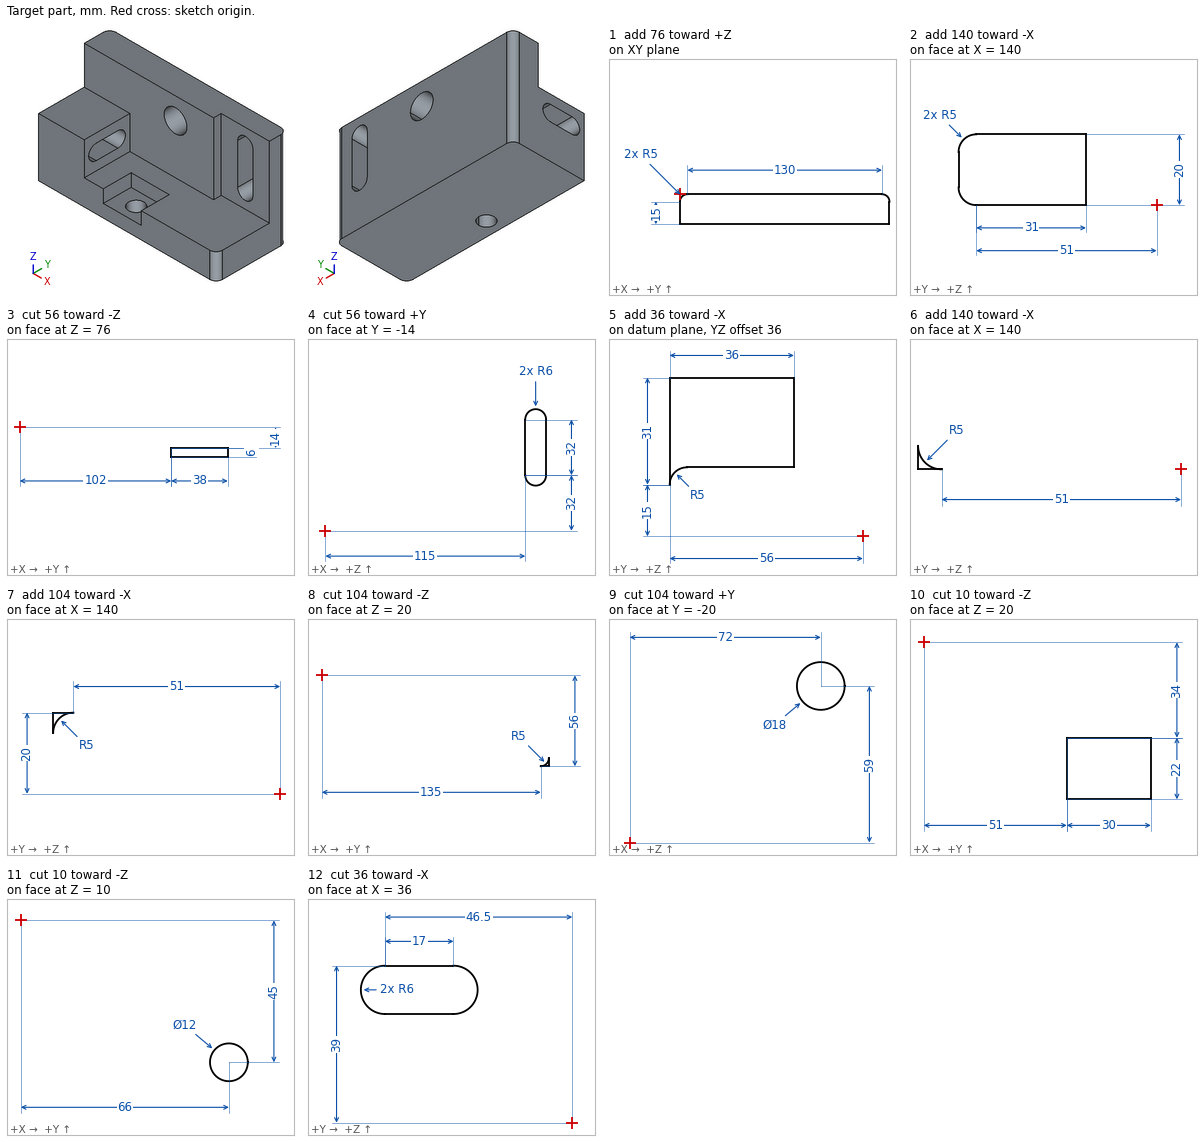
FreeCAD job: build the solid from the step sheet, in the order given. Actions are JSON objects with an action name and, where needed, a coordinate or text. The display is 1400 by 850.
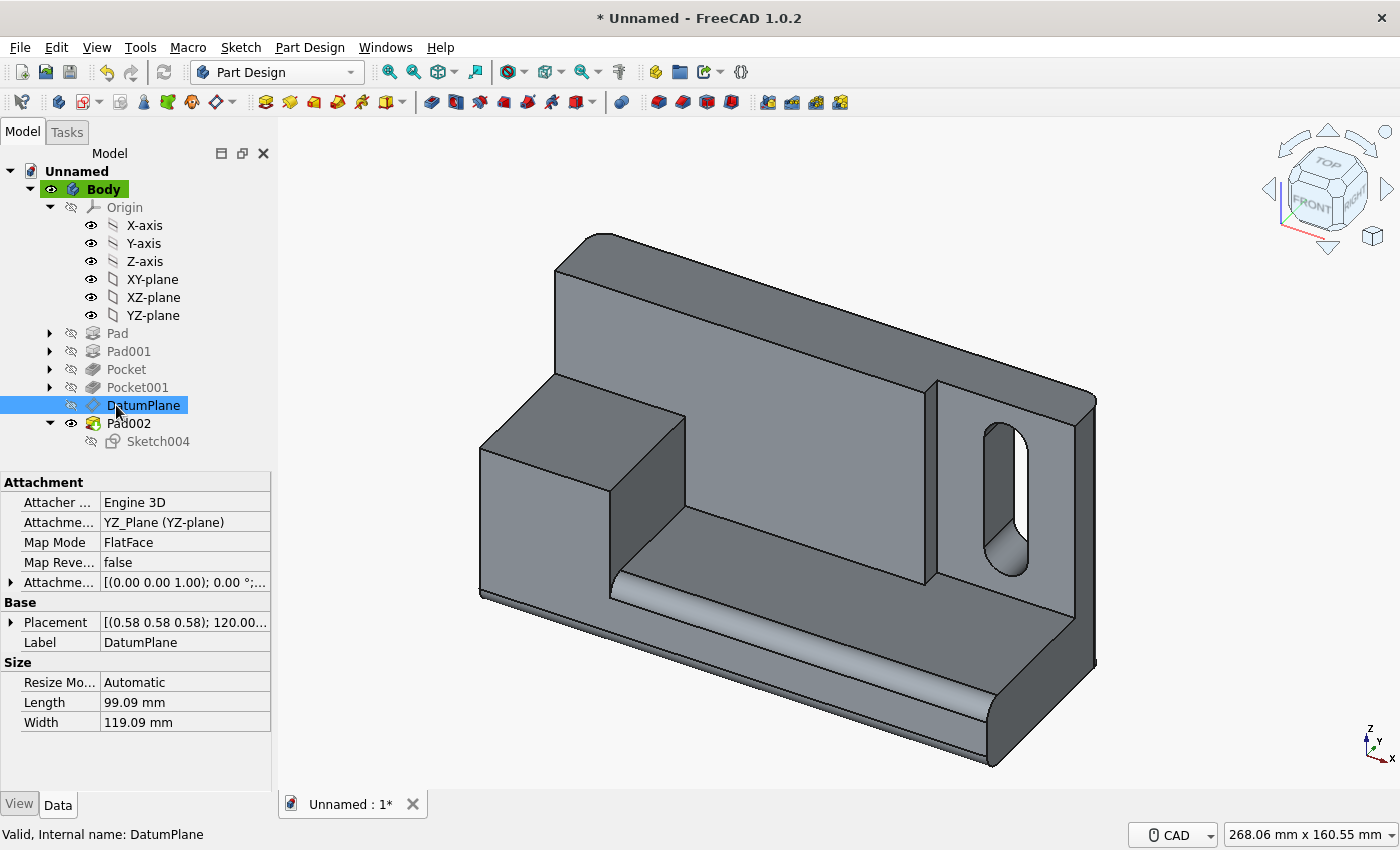
{"action": "left_click", "coordinate": [1071, 671]}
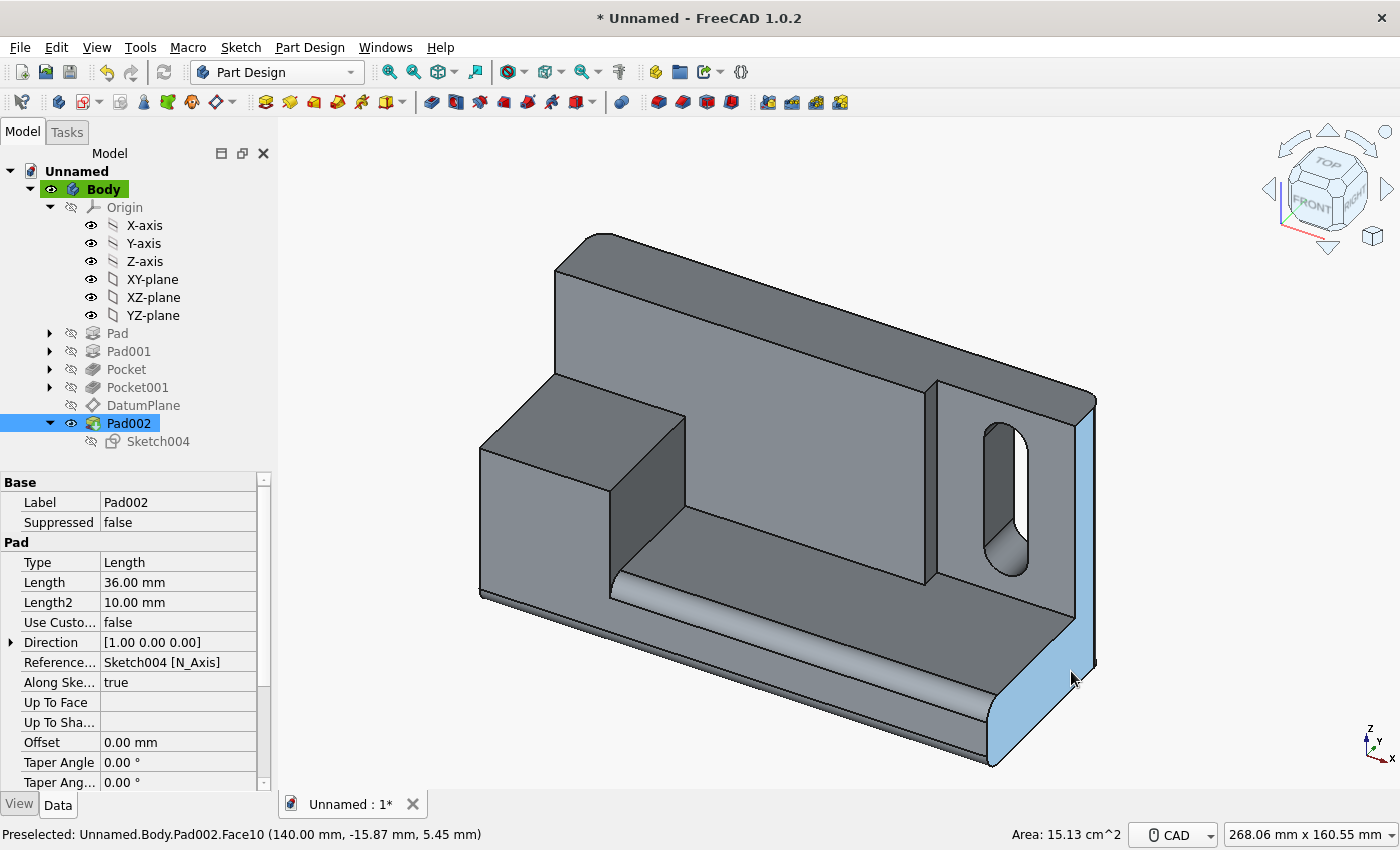
{"action": "left_click", "coordinate": [84, 102]}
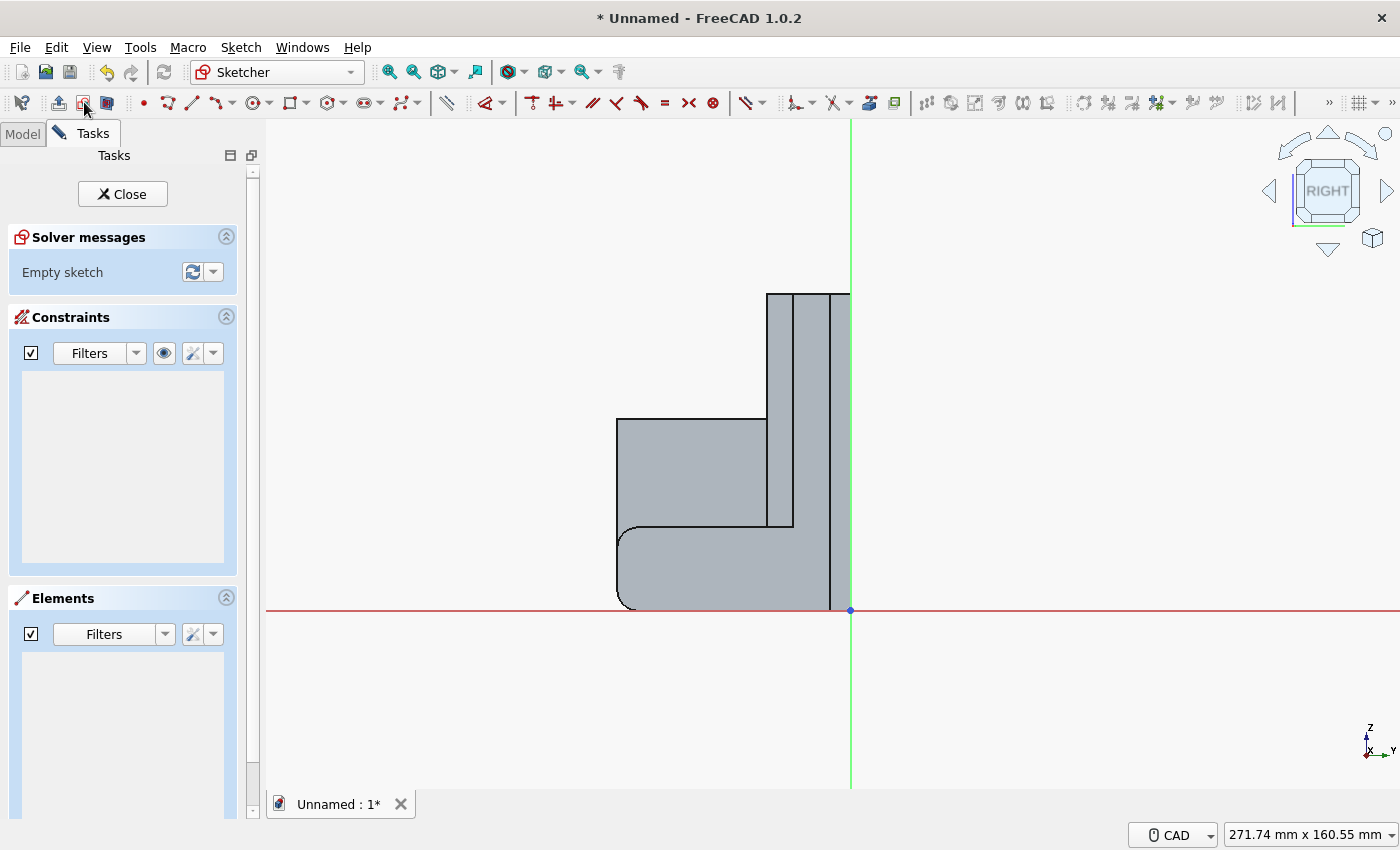
{"action": "scroll", "coordinate": [621, 608], "scroll_direction": "up", "scroll_amount": 15}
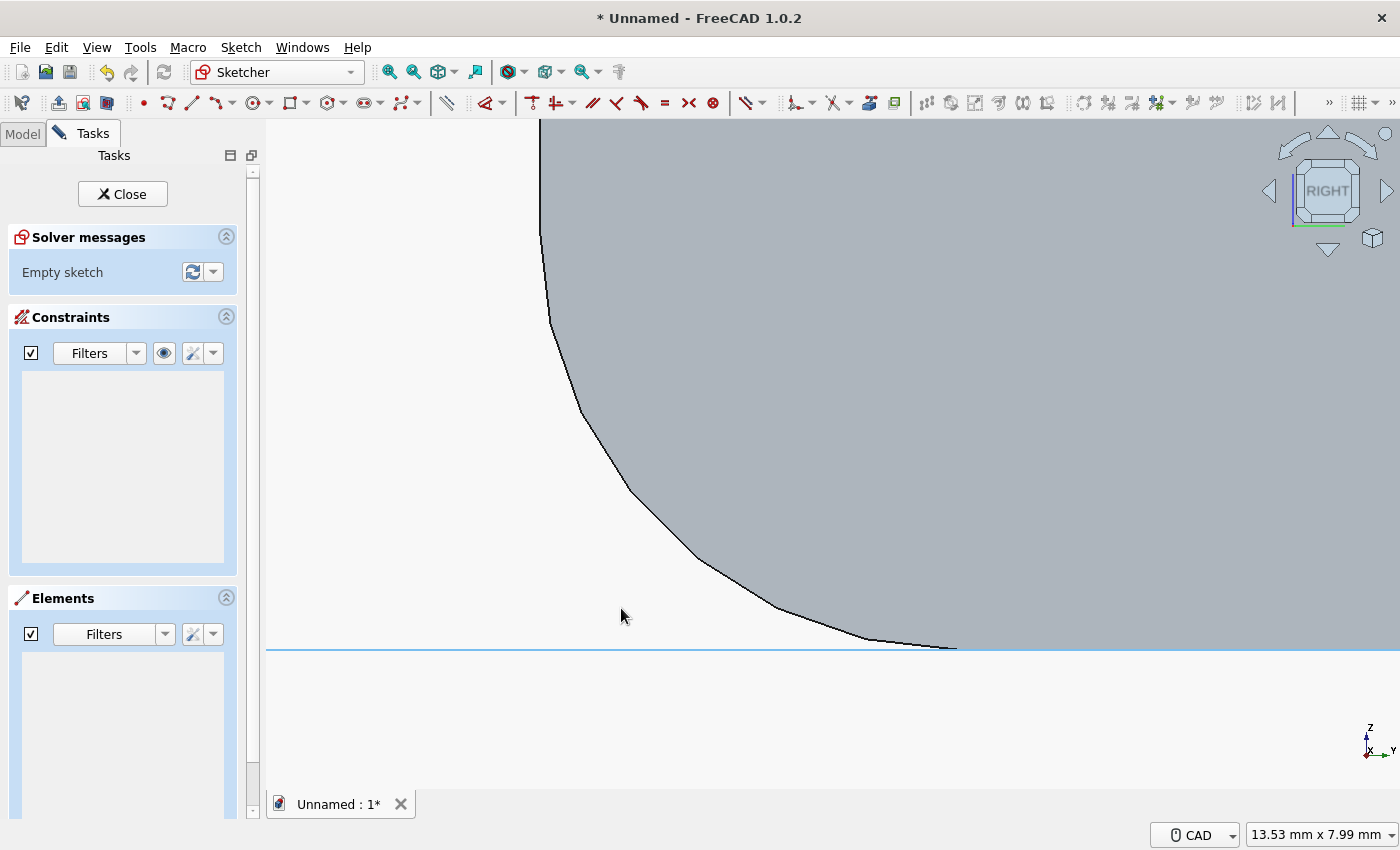
{"action": "left_click", "coordinate": [168, 104]}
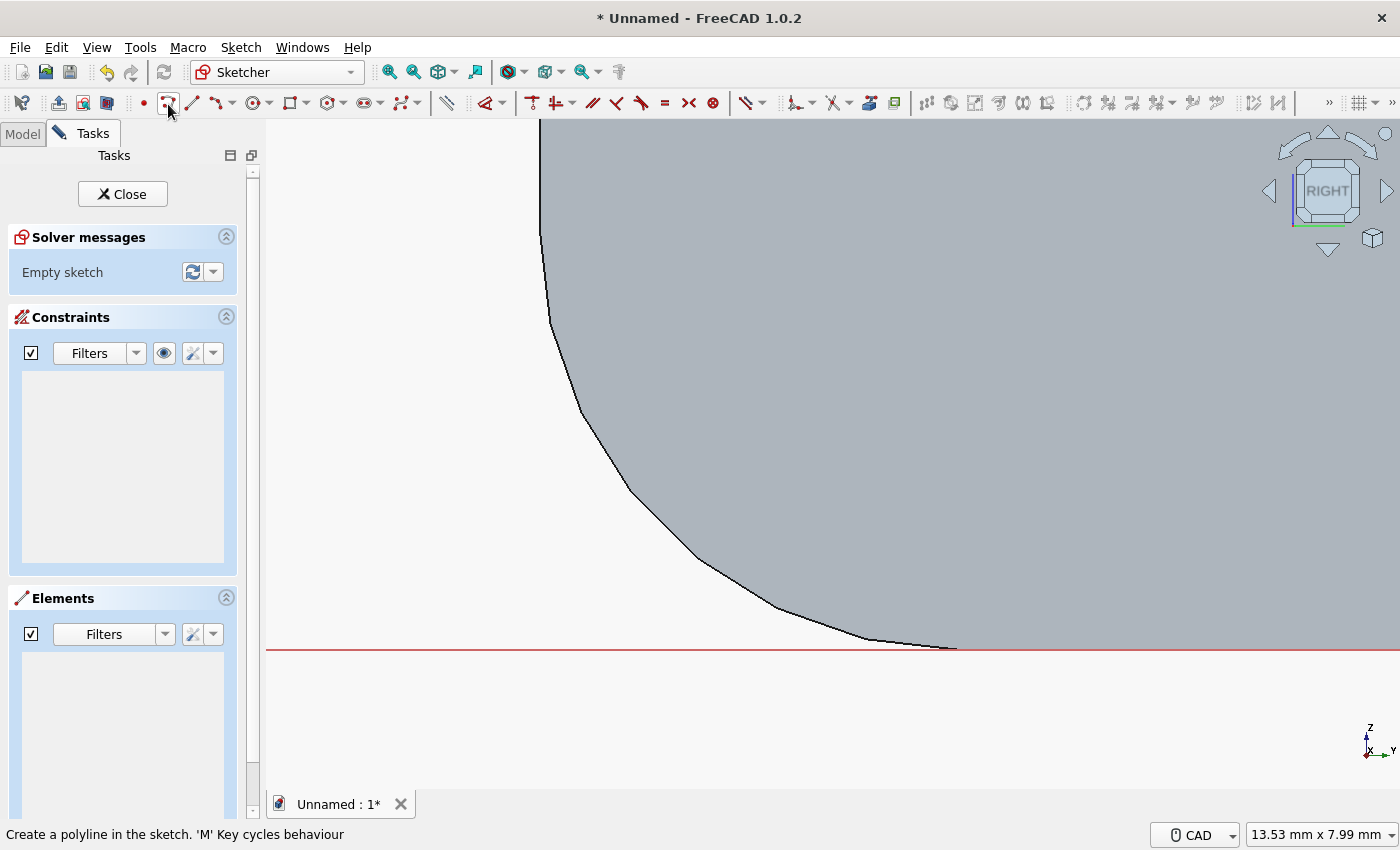
{"action": "left_click", "coordinate": [959, 650]}
{"action": "left_click", "coordinate": [540, 641]}
{"action": "left_click", "coordinate": [540, 231]}
{"action": "right_click", "coordinate": [540, 231]}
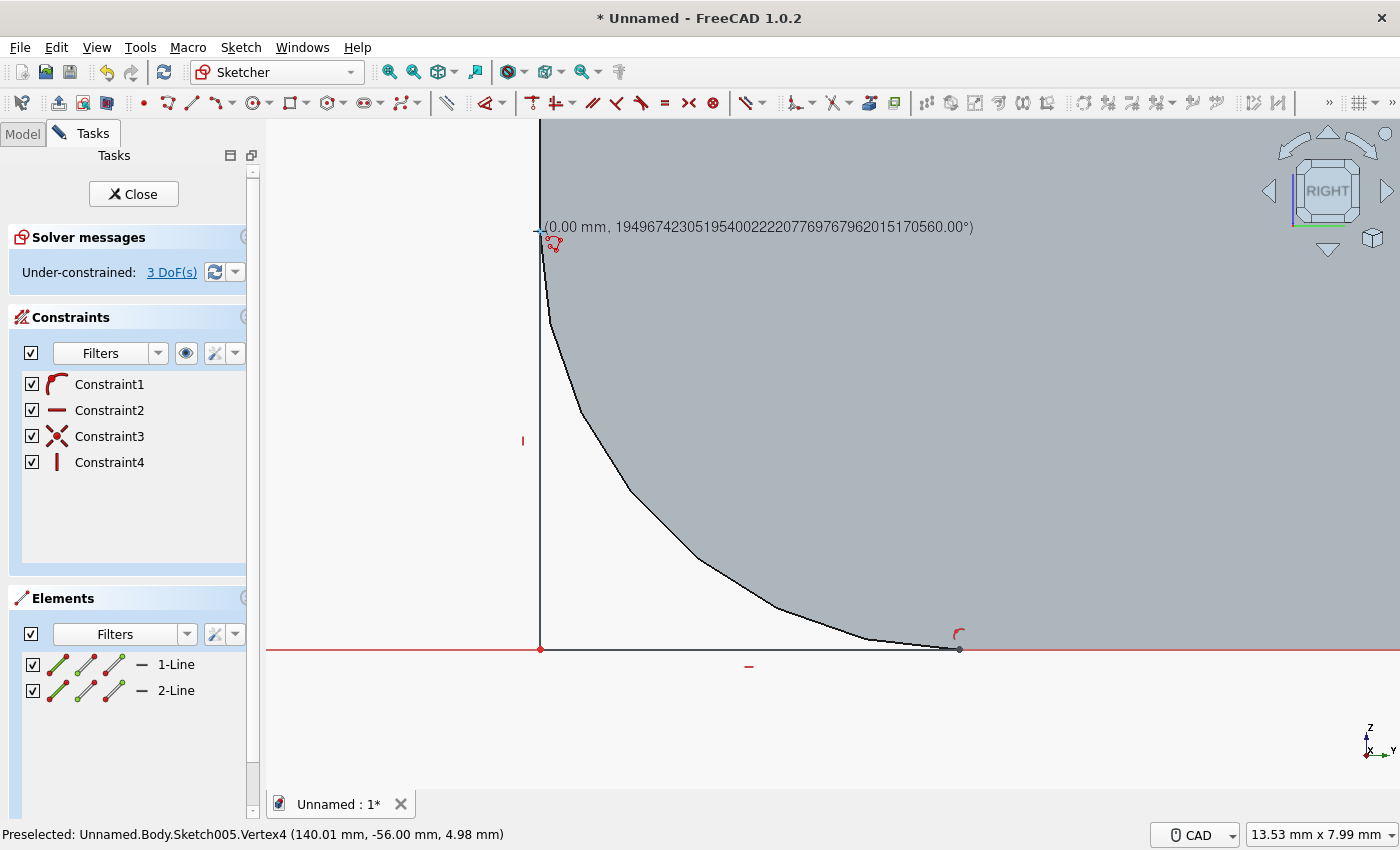
{"action": "key", "text": "g 3 a"}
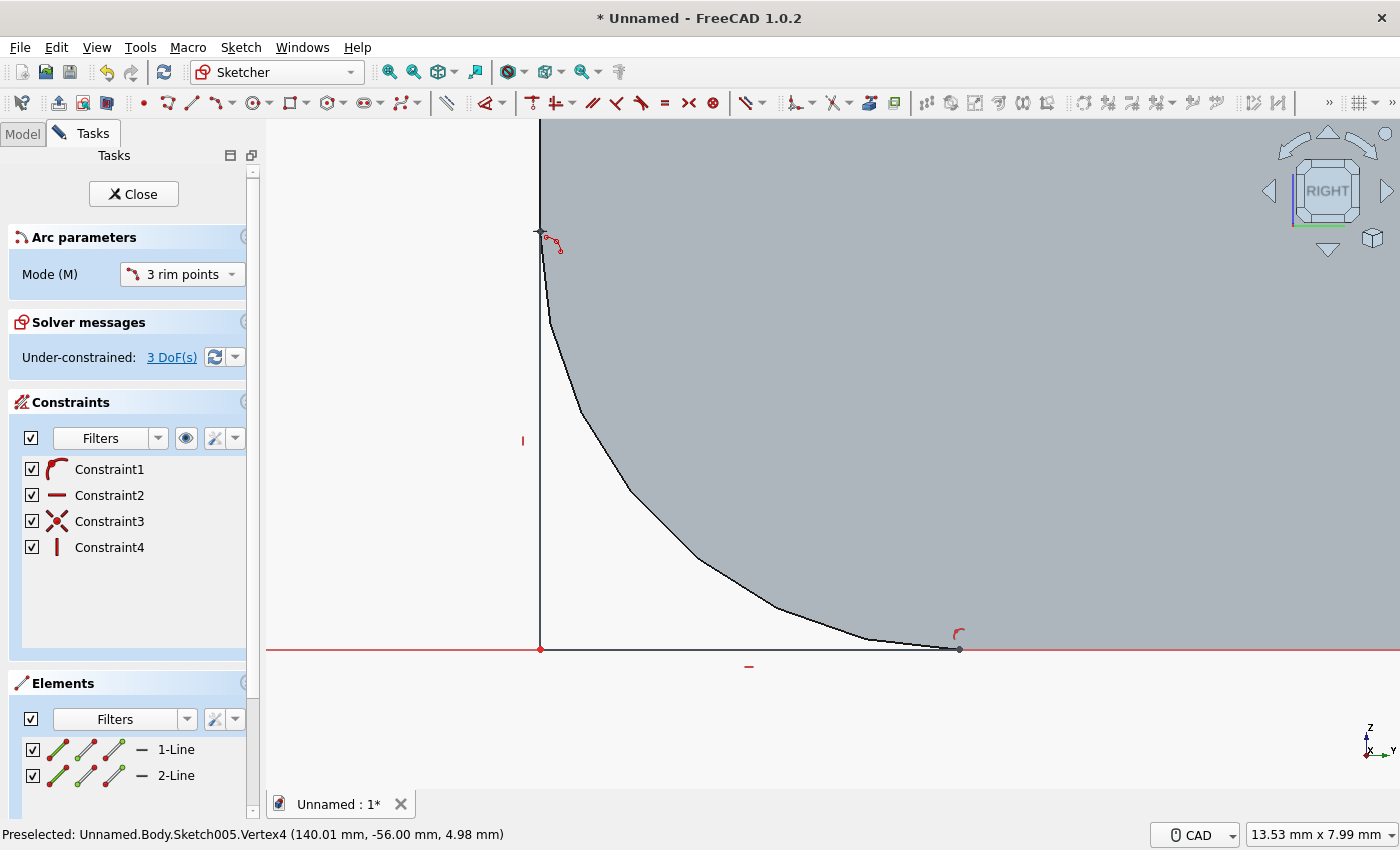
{"action": "left_click", "coordinate": [540, 232]}
{"action": "left_click", "coordinate": [959, 650]}
{"action": "left_click", "coordinate": [663, 527]}
{"action": "key", "text": "Escape"}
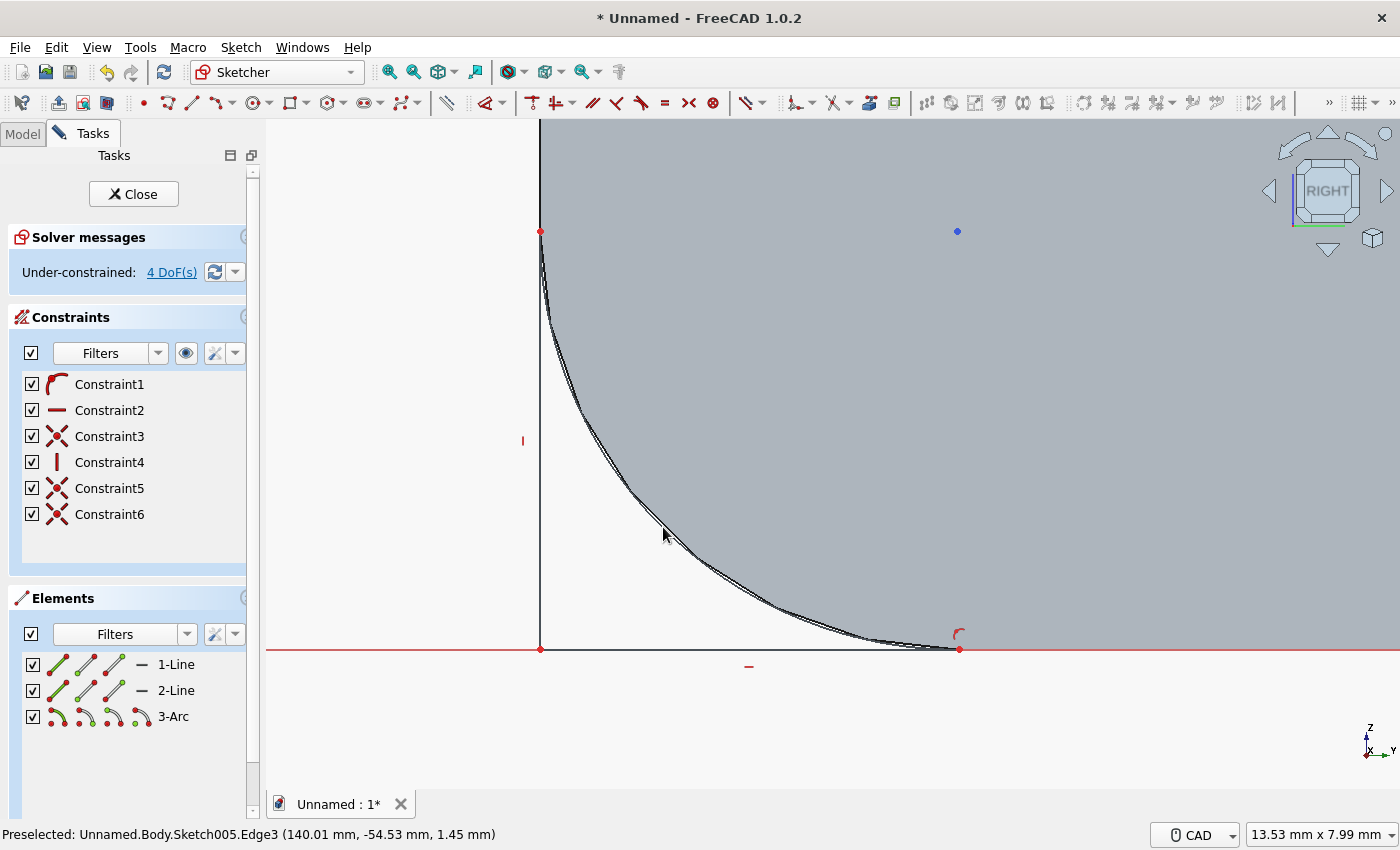
{"action": "left_click", "coordinate": [833, 650]}